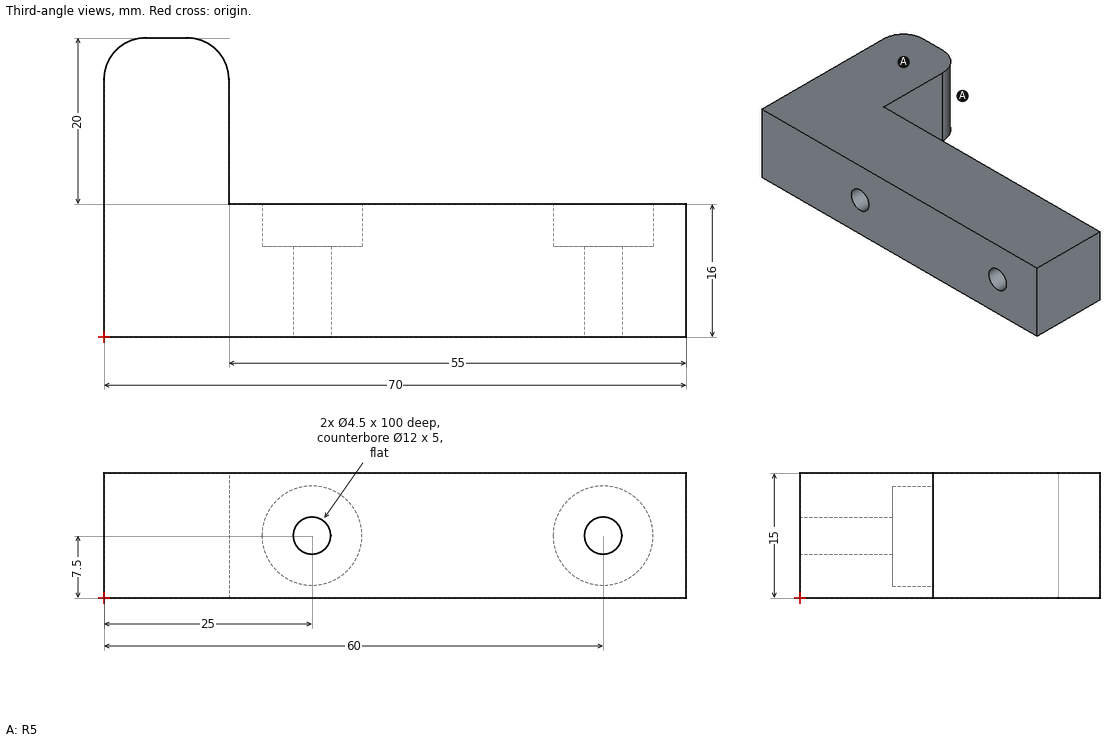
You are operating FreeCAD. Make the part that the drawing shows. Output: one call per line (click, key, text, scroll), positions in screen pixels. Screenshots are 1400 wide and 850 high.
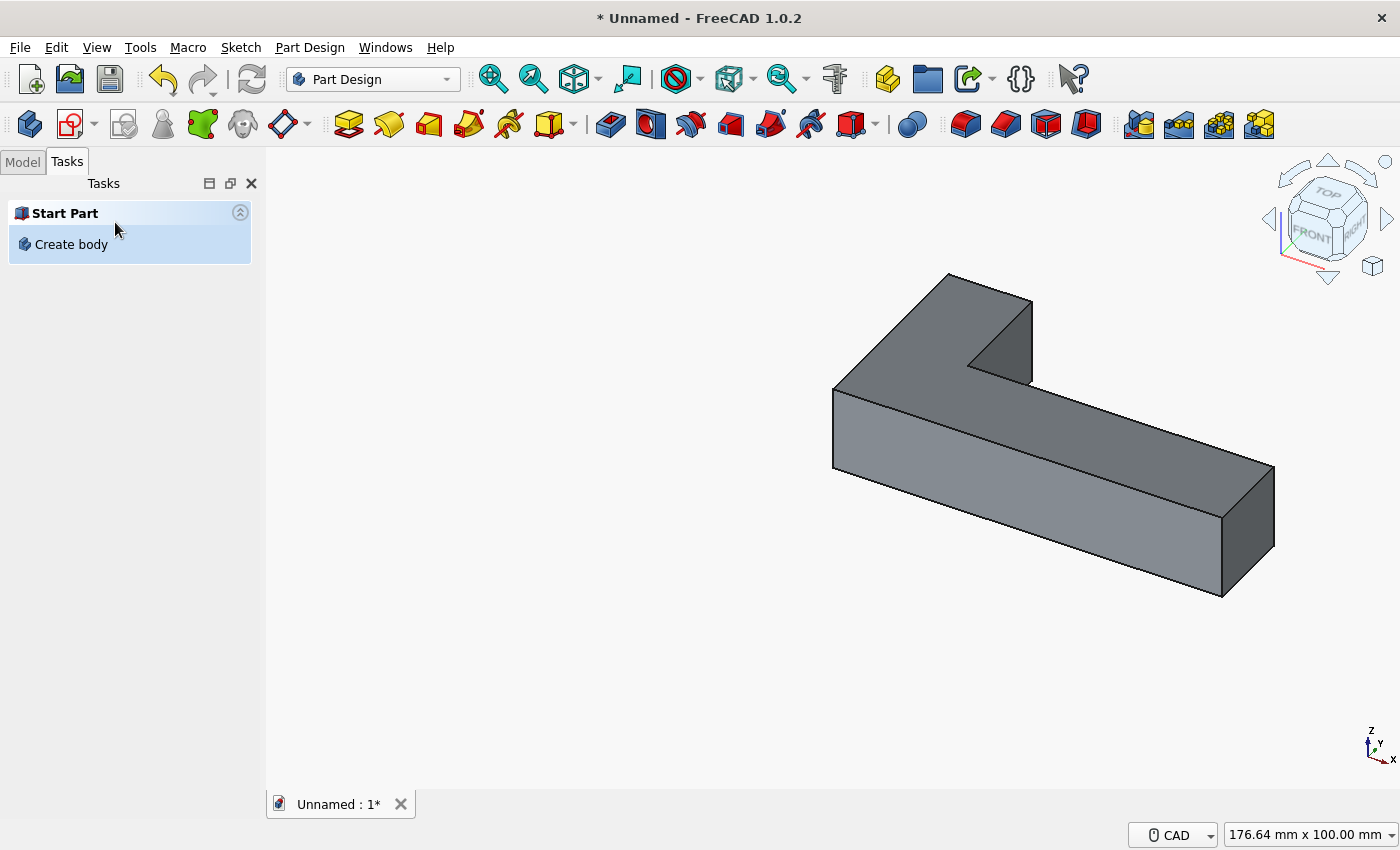
key(0)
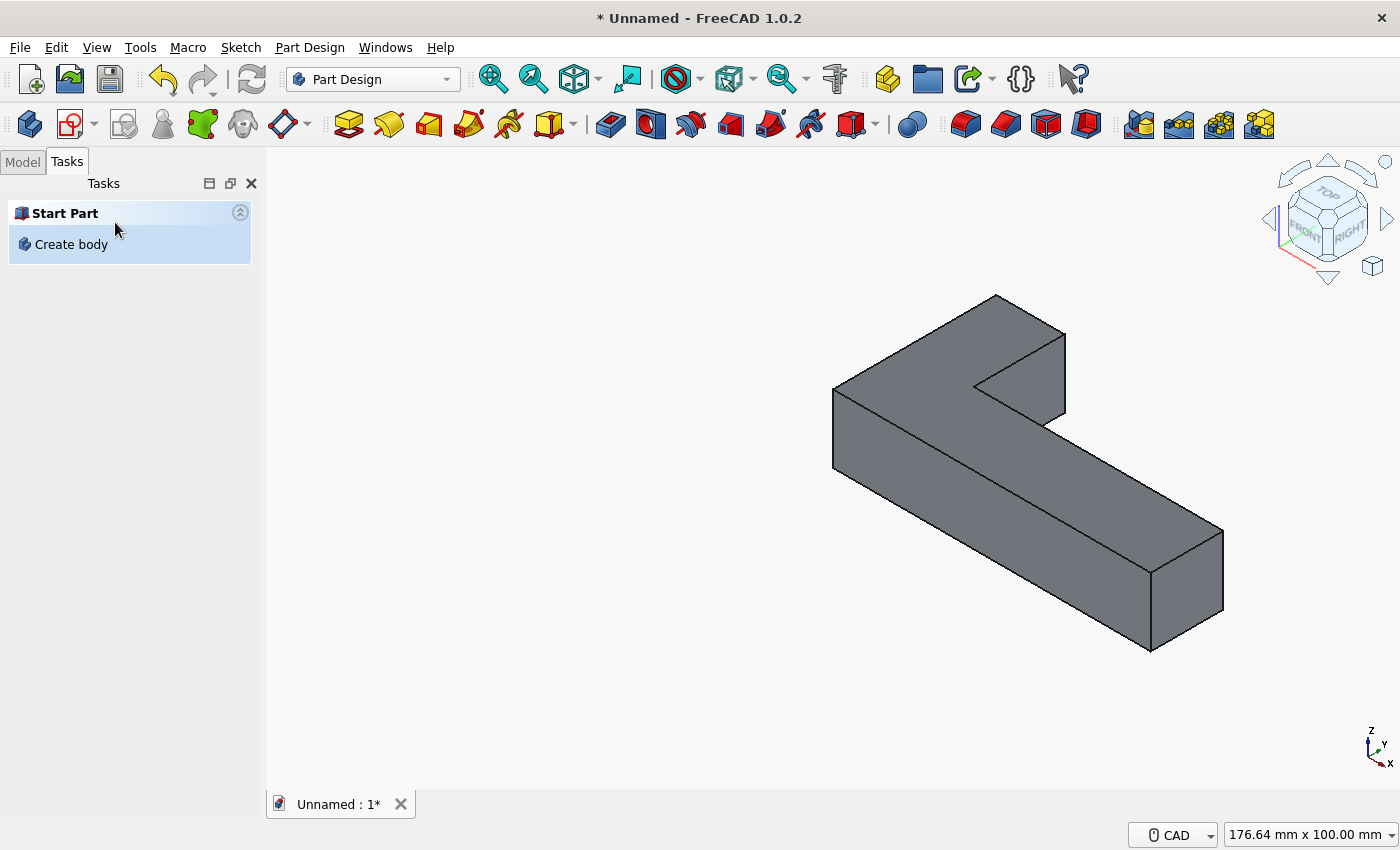
key(2)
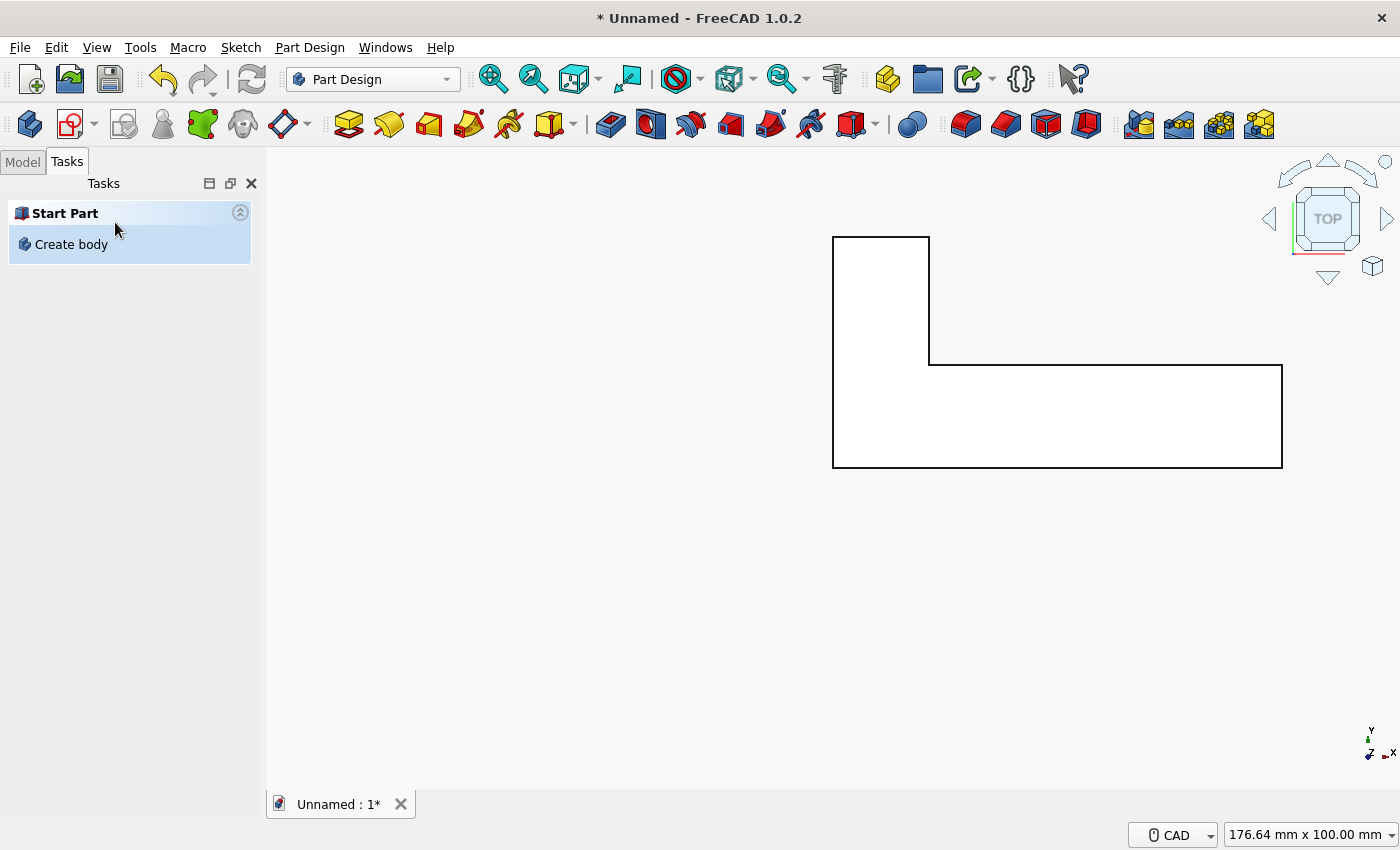
click(494, 80)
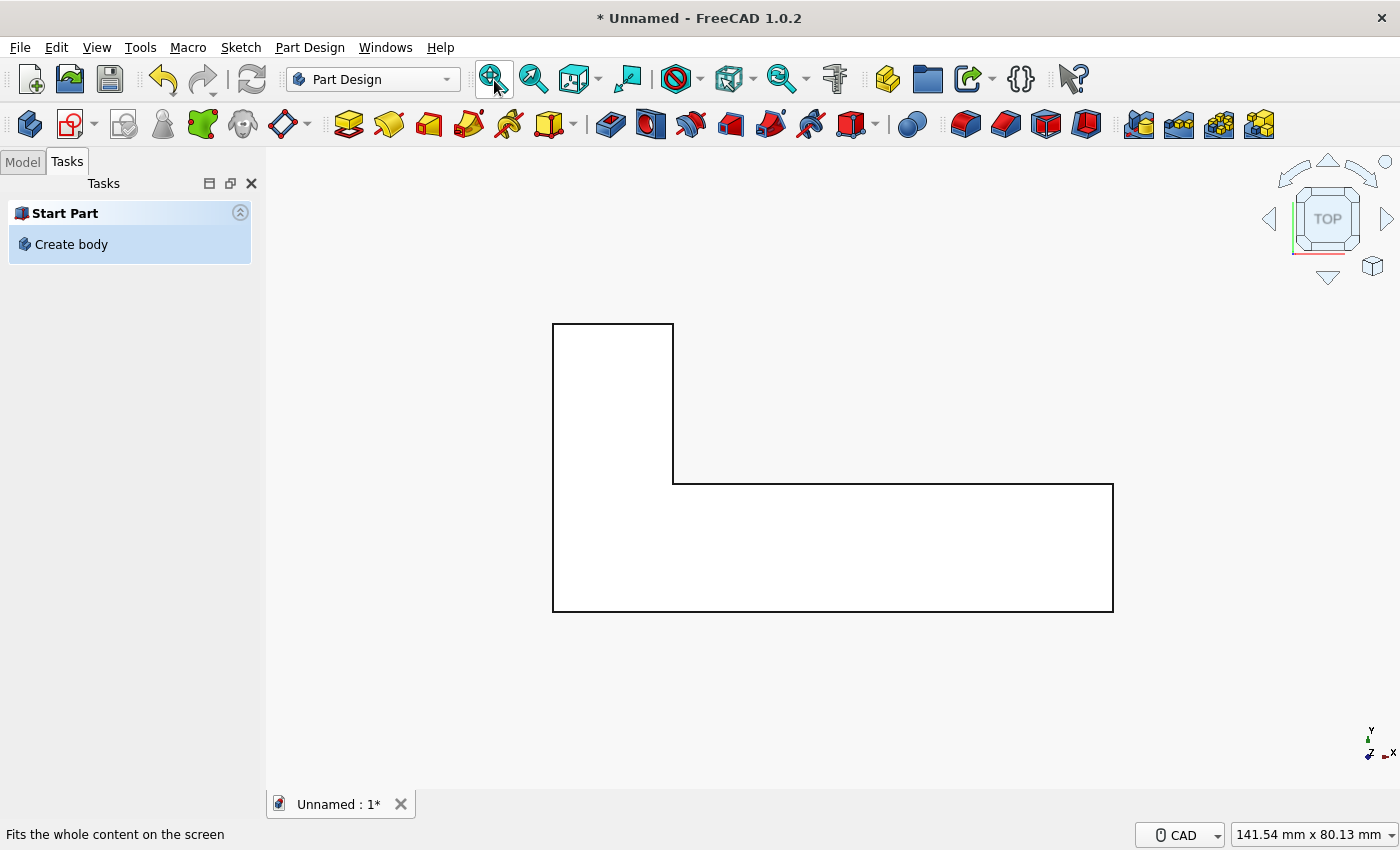
key(1)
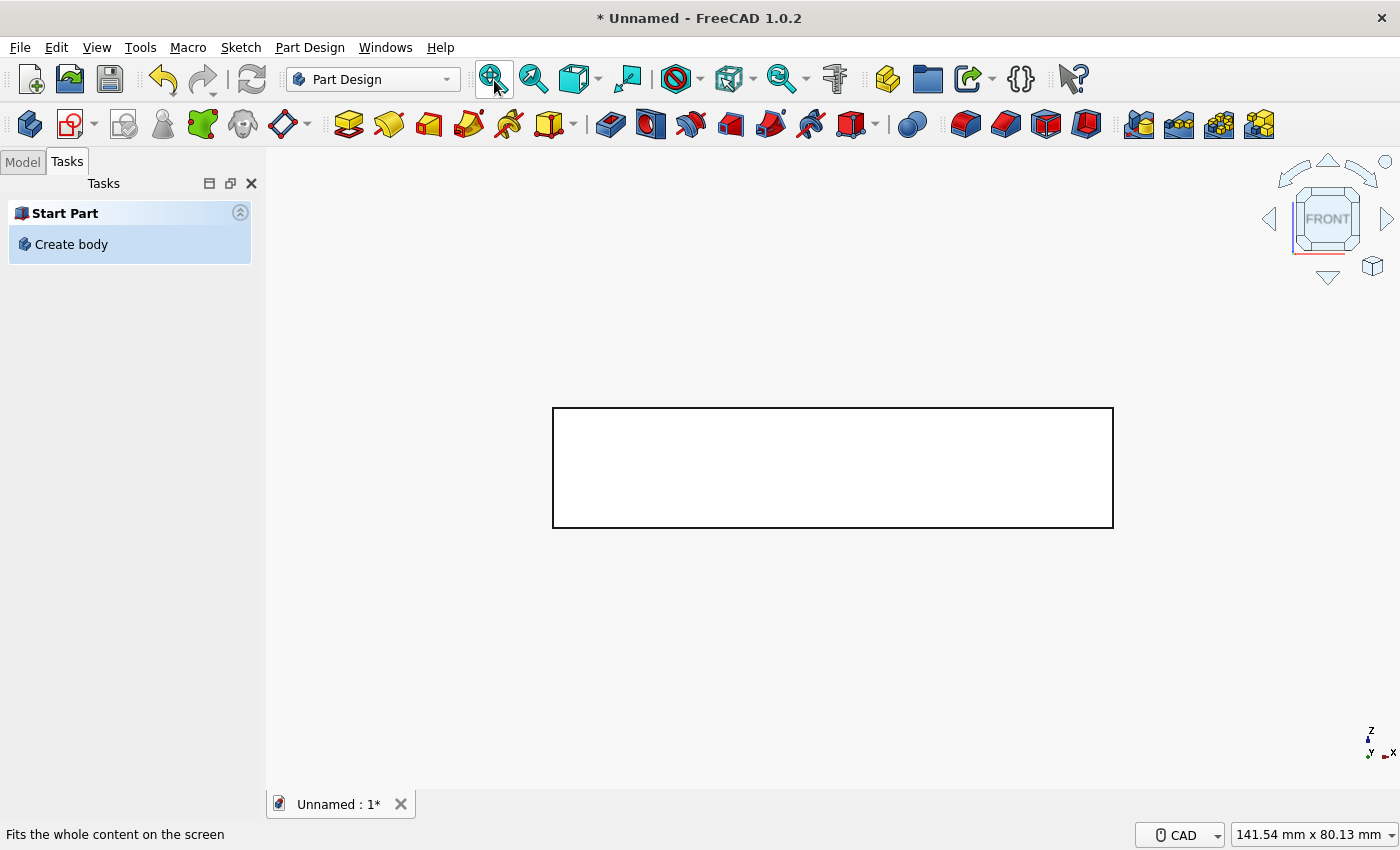
key(3)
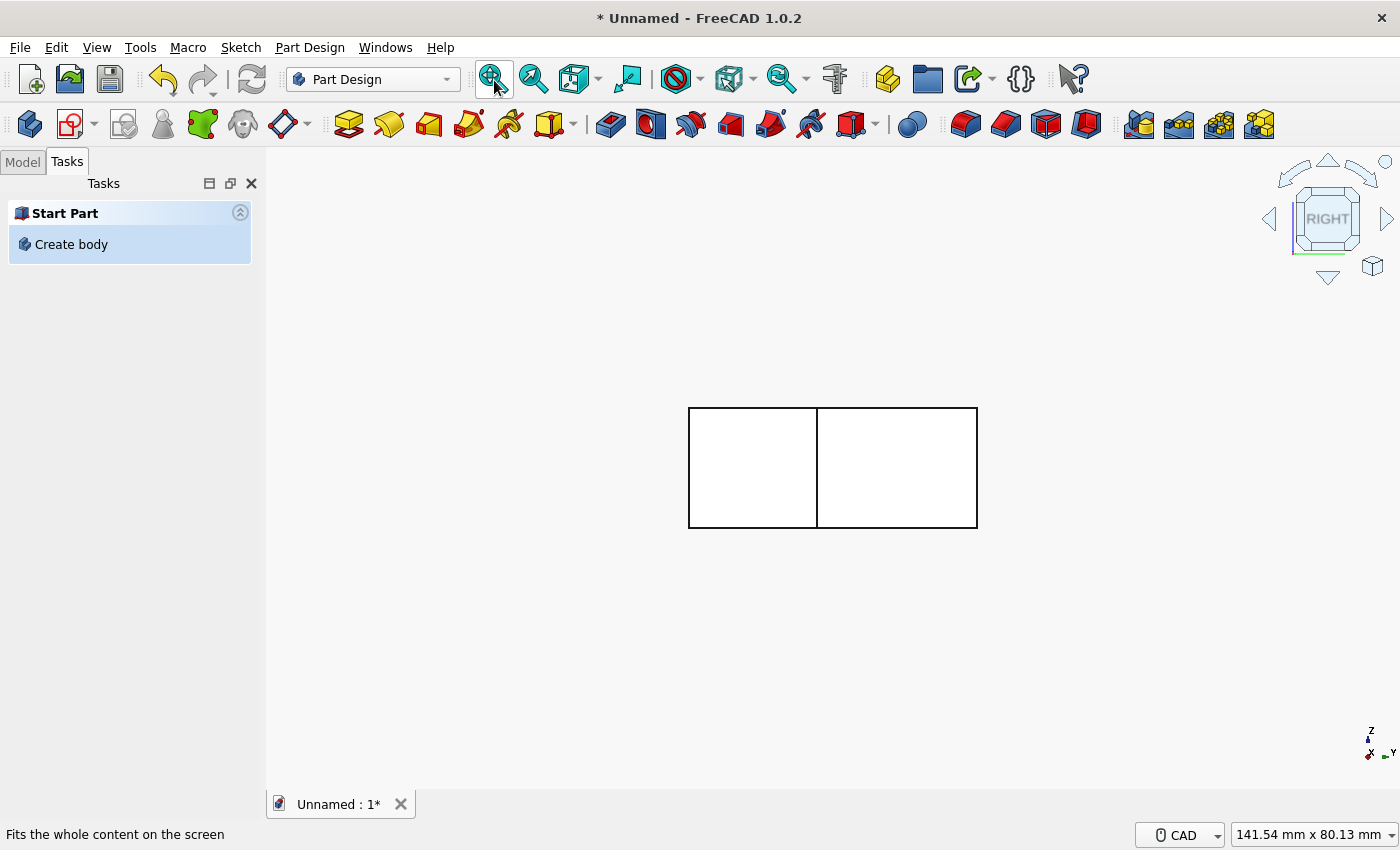
click(494, 80)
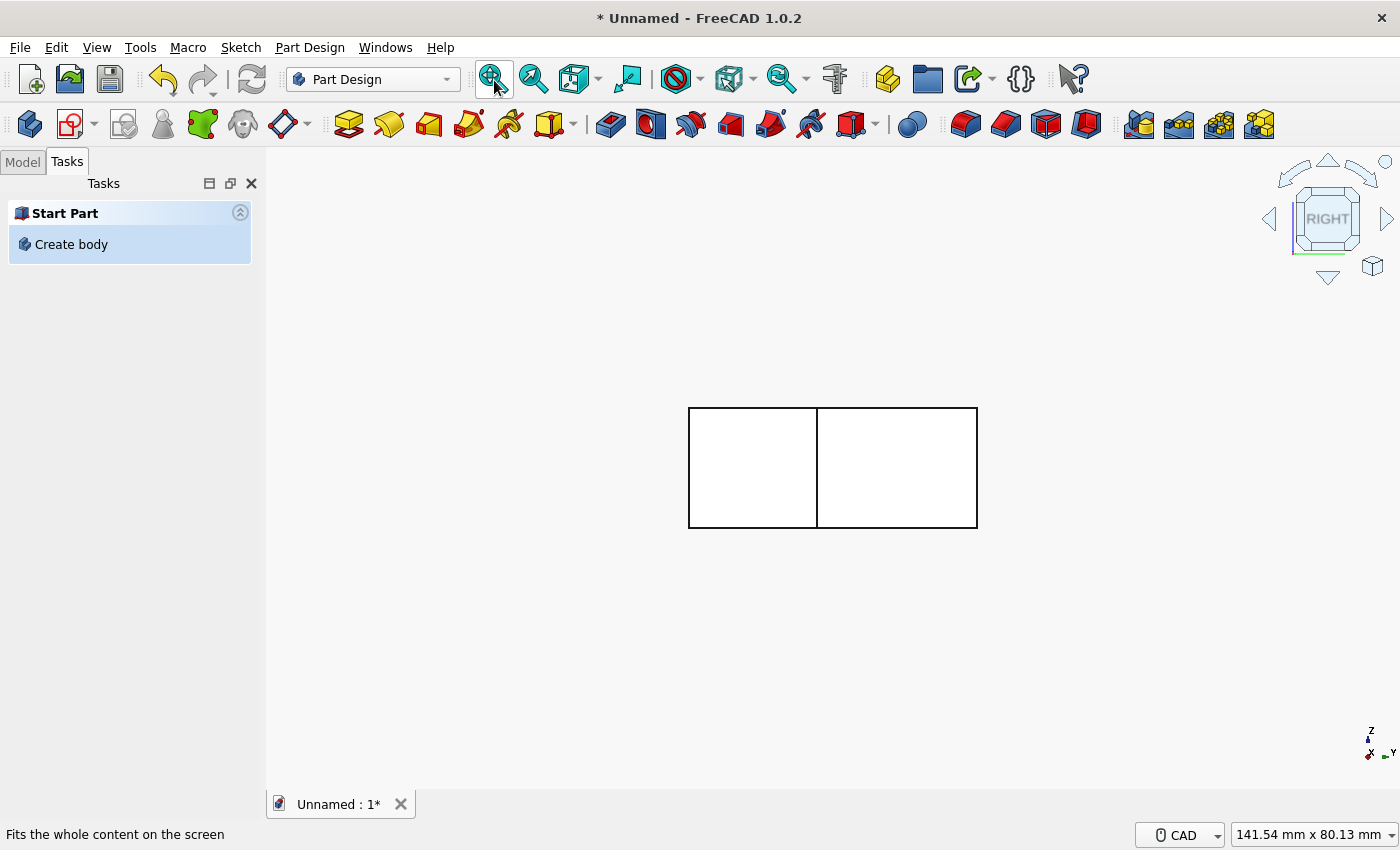
click(977, 467)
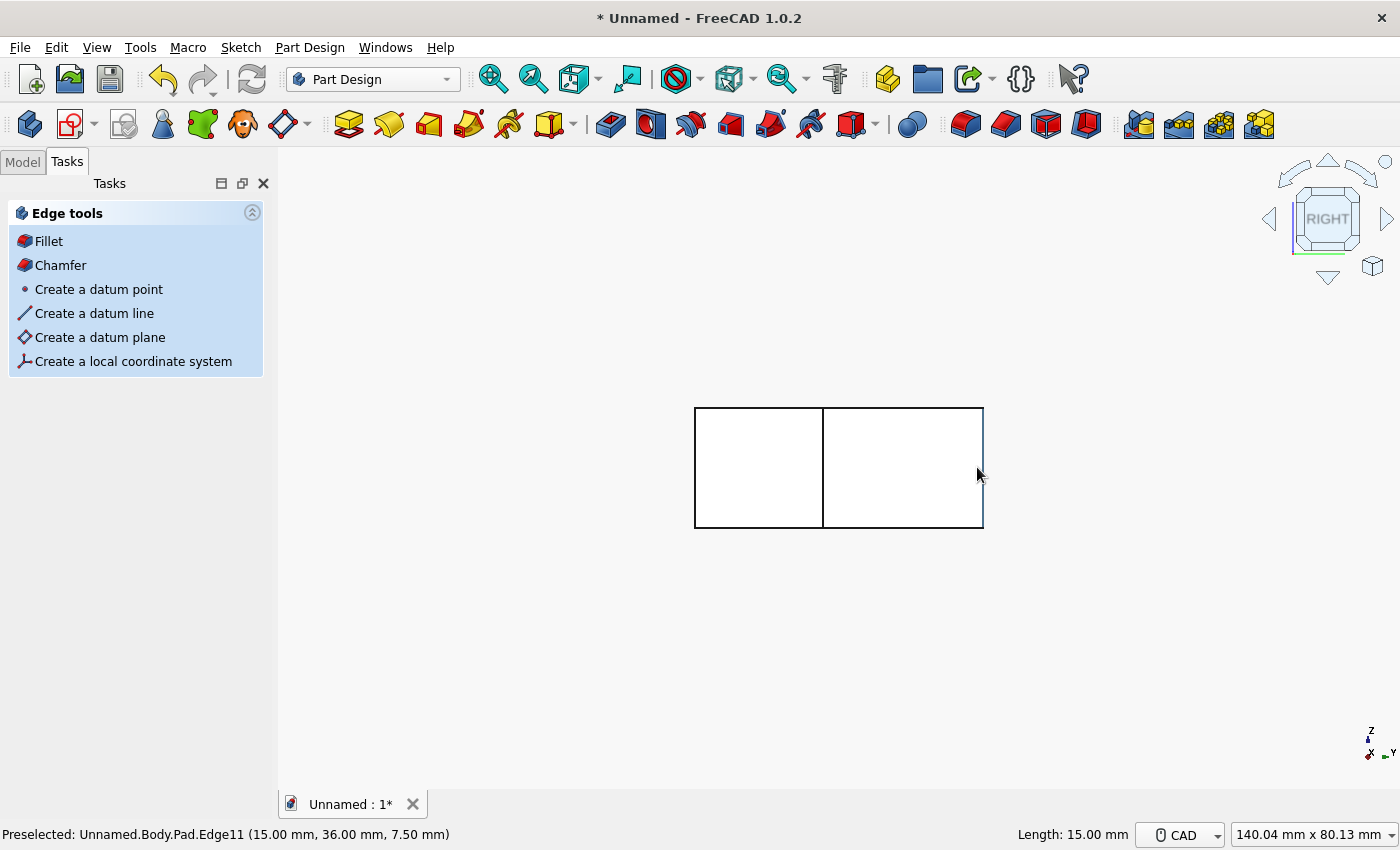
key(5)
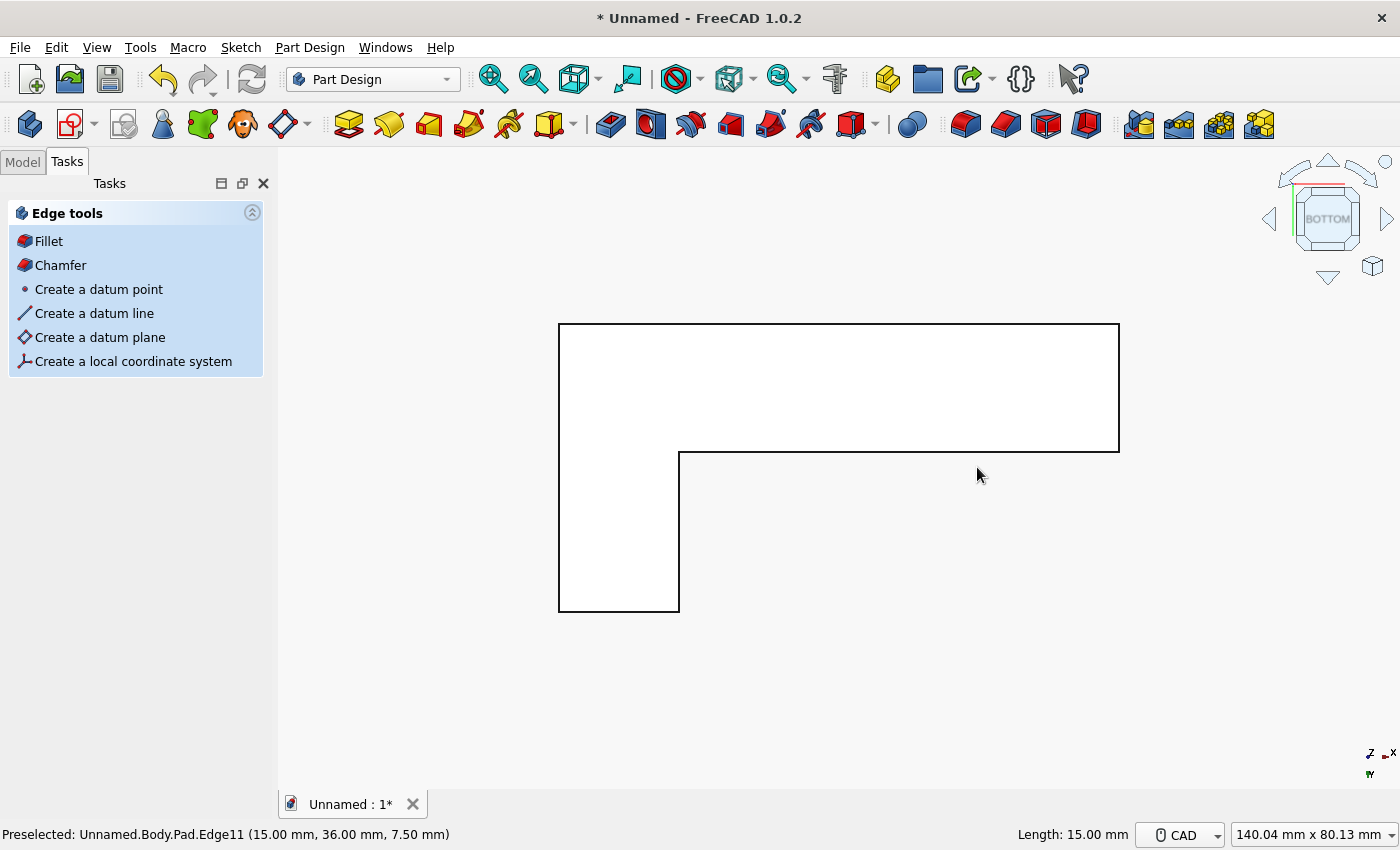
key(4)